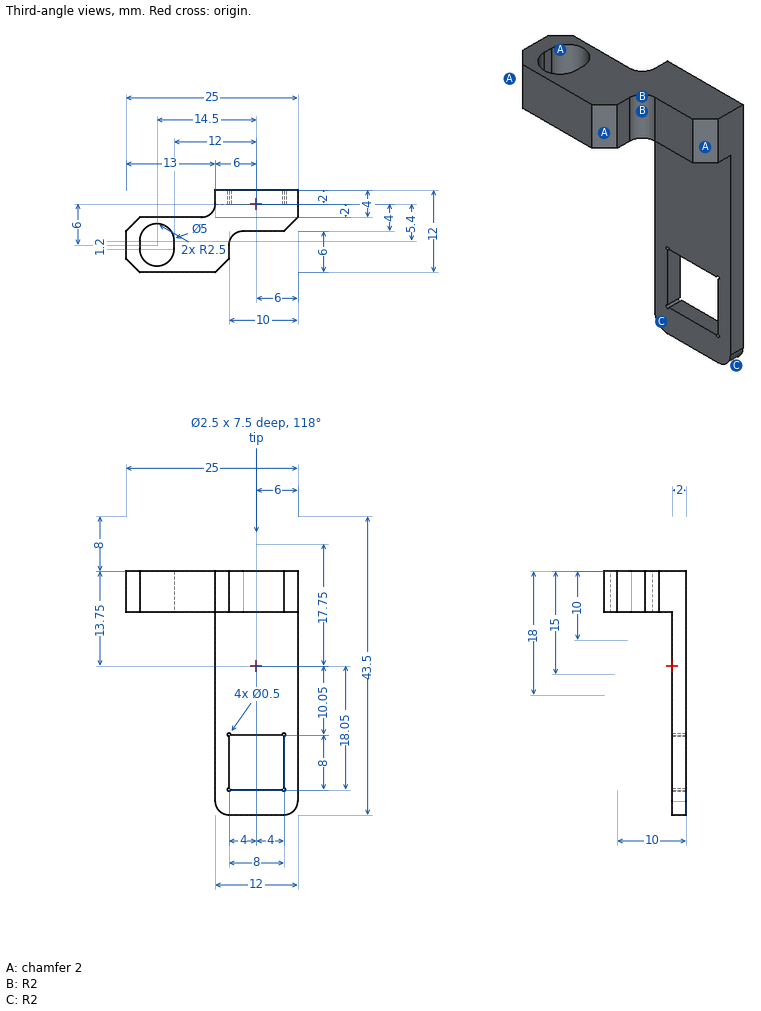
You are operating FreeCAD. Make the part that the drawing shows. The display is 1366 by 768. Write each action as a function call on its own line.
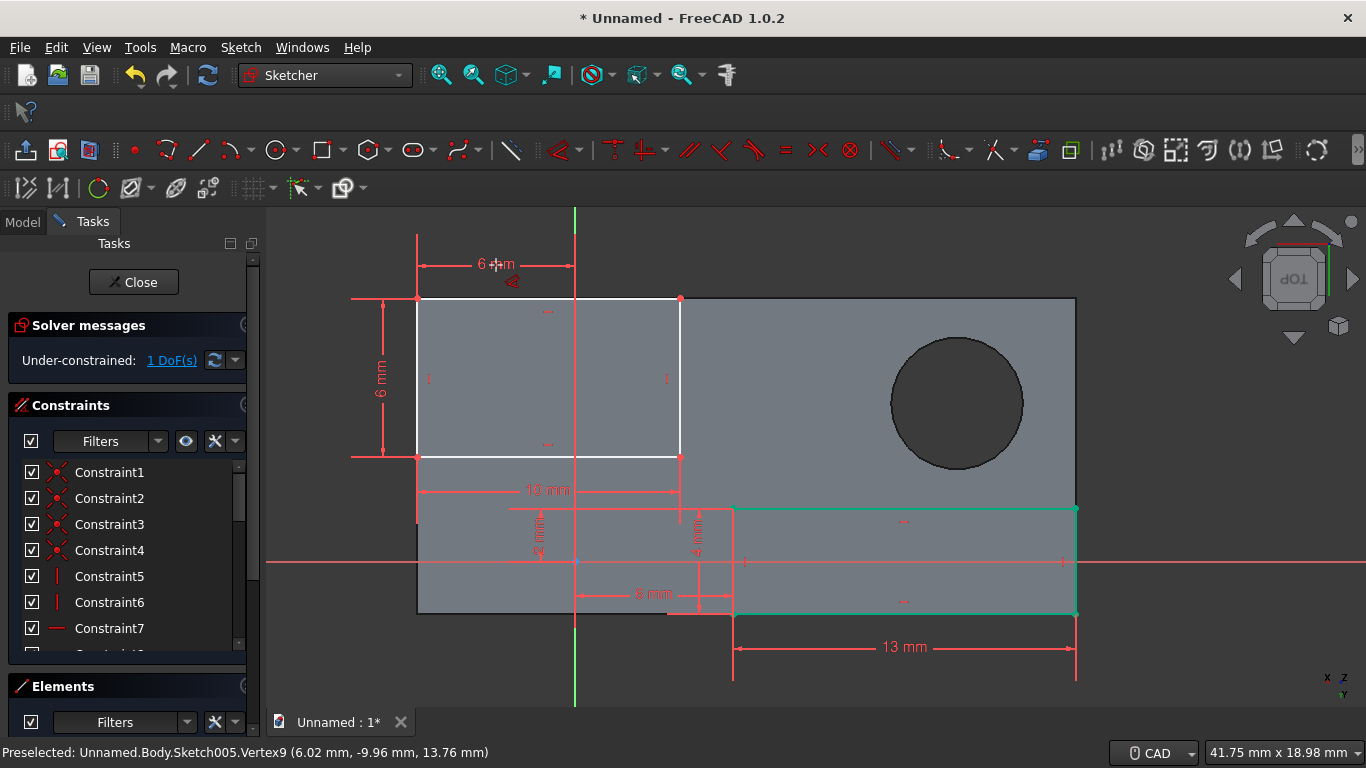
click(417, 457)
click(383, 509)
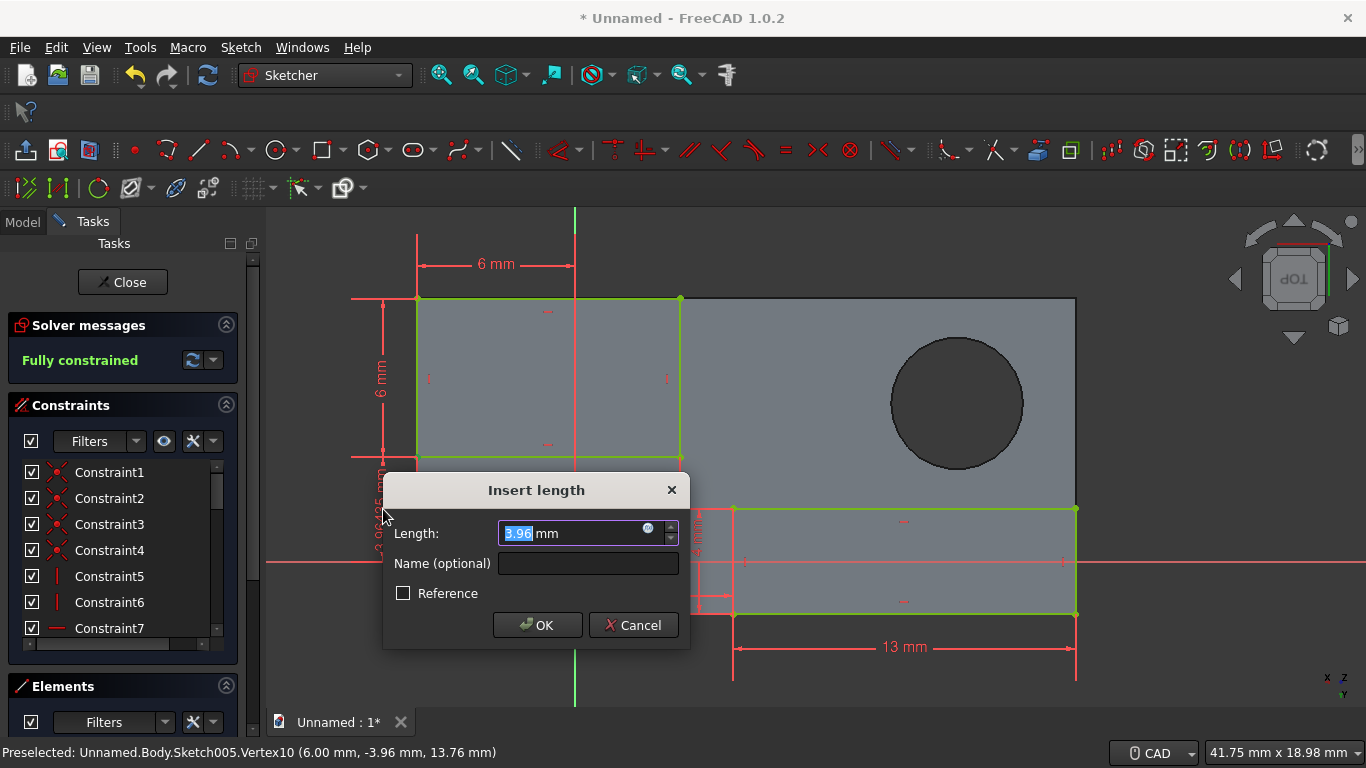
text(4)
key(Return)
key(Escape)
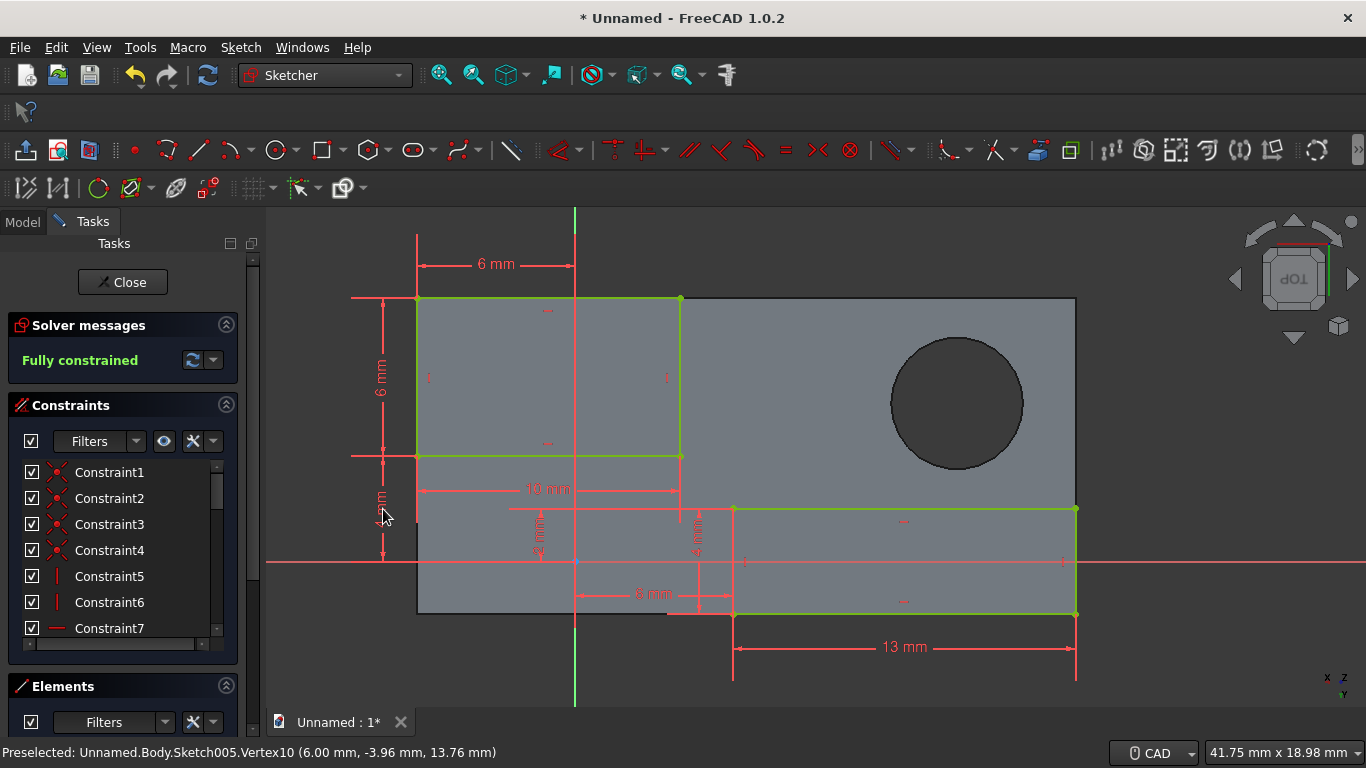
click(123, 282)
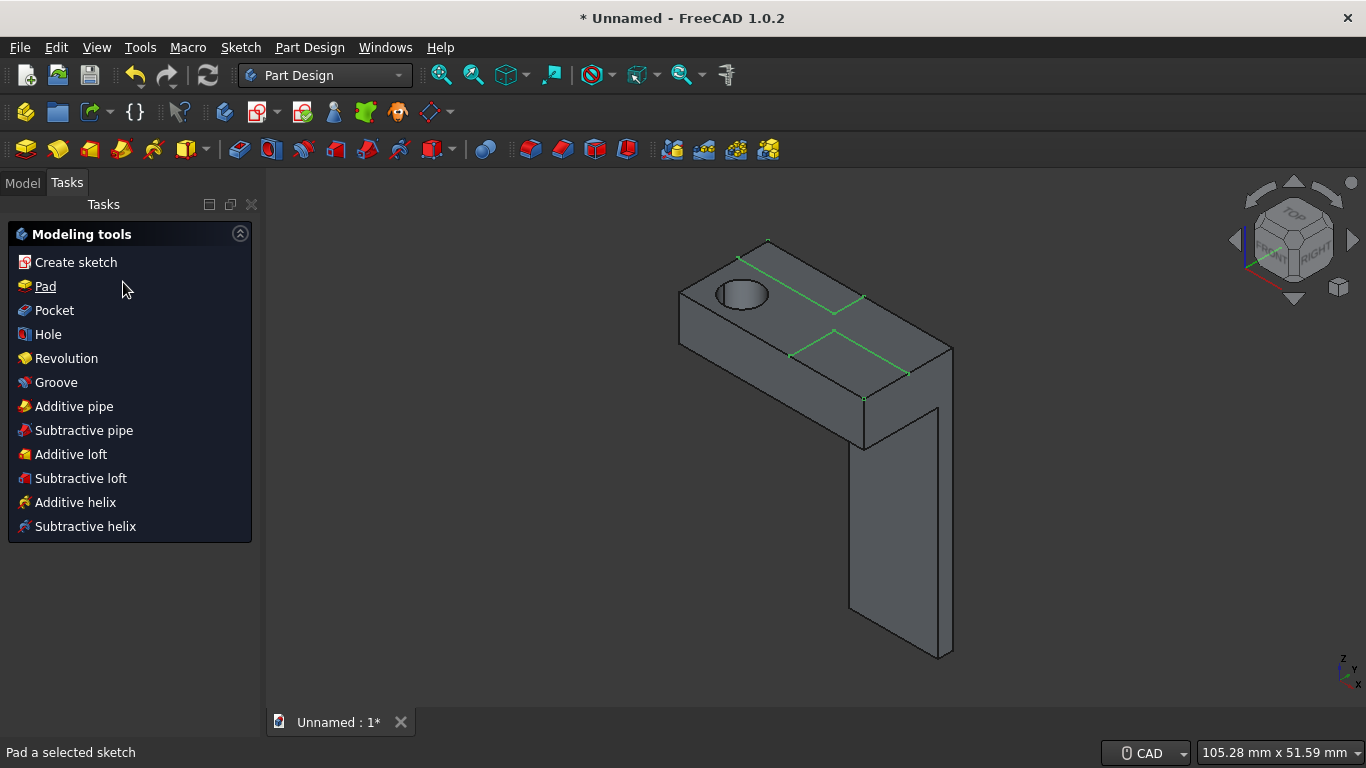
click(240, 150)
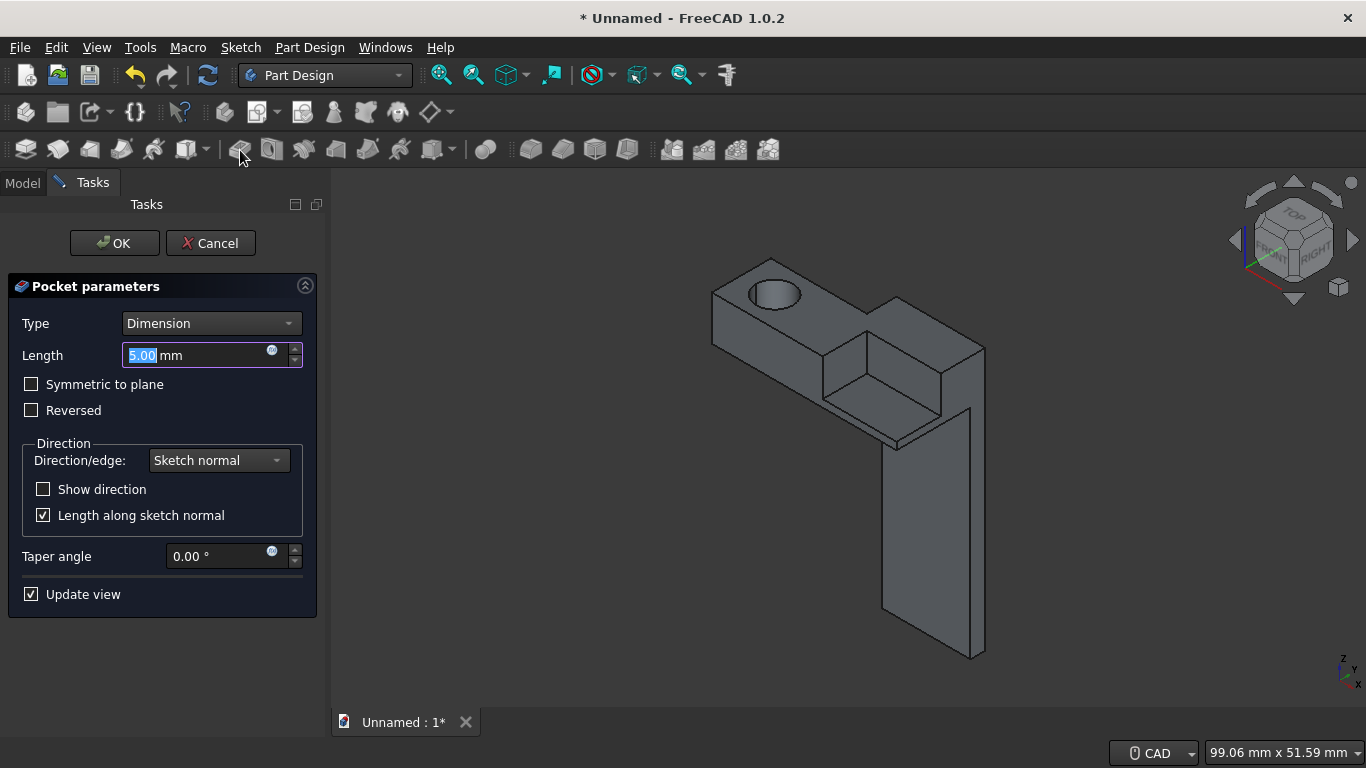
text(18)
key(Tab)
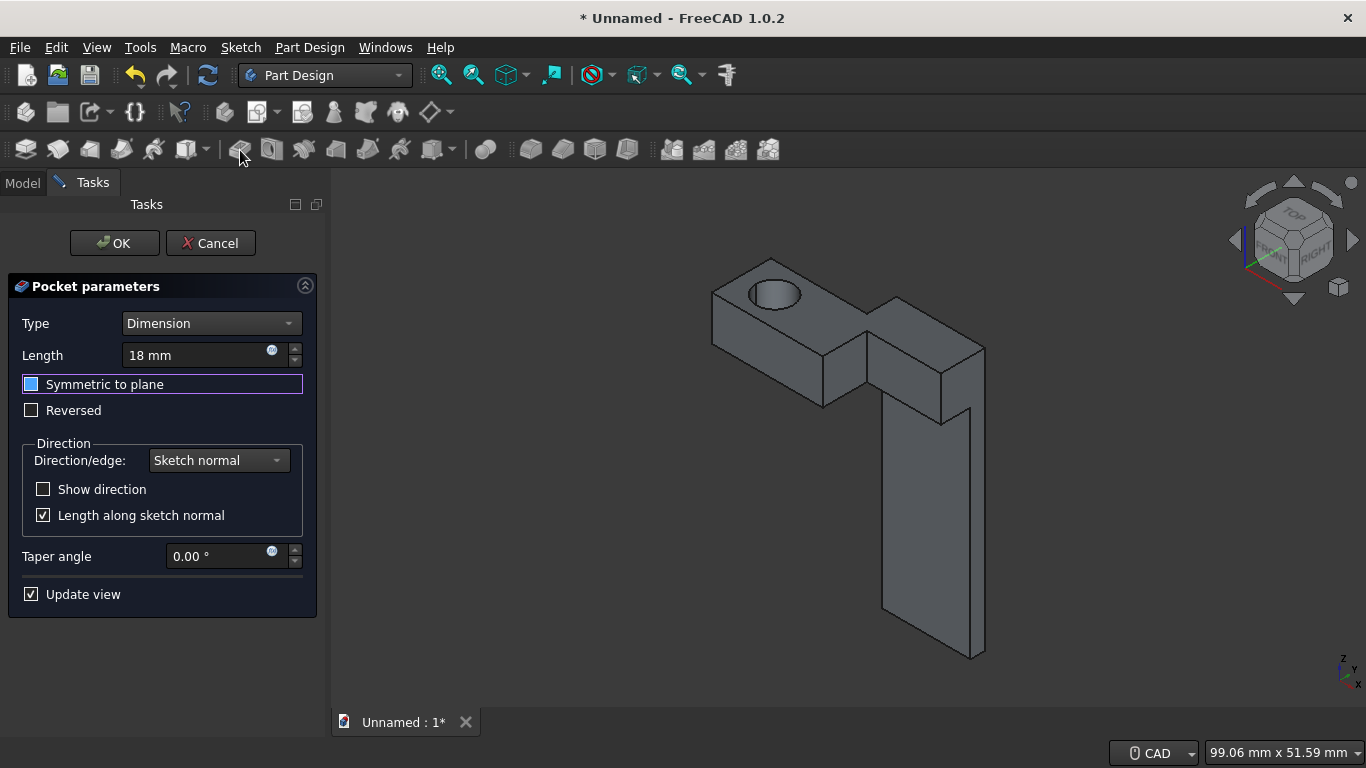
click(115, 243)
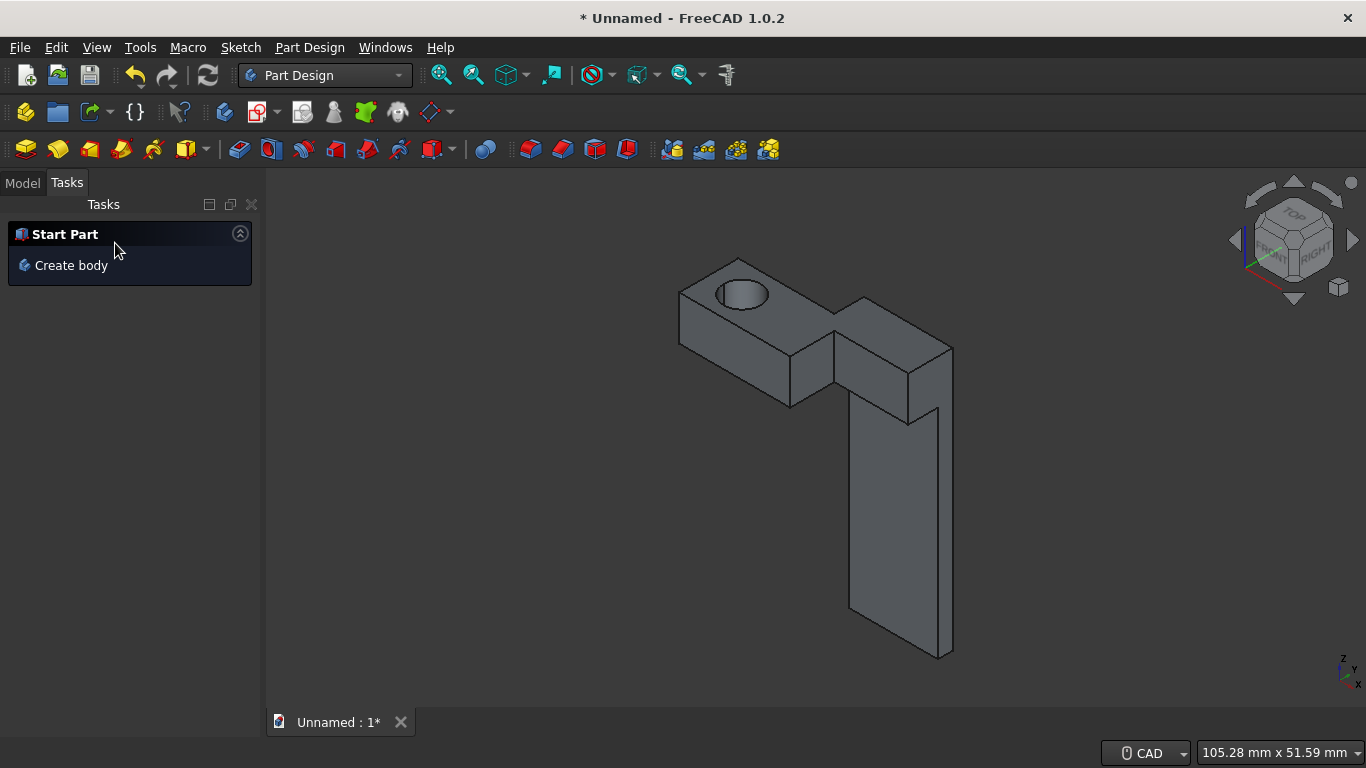
click(908, 398)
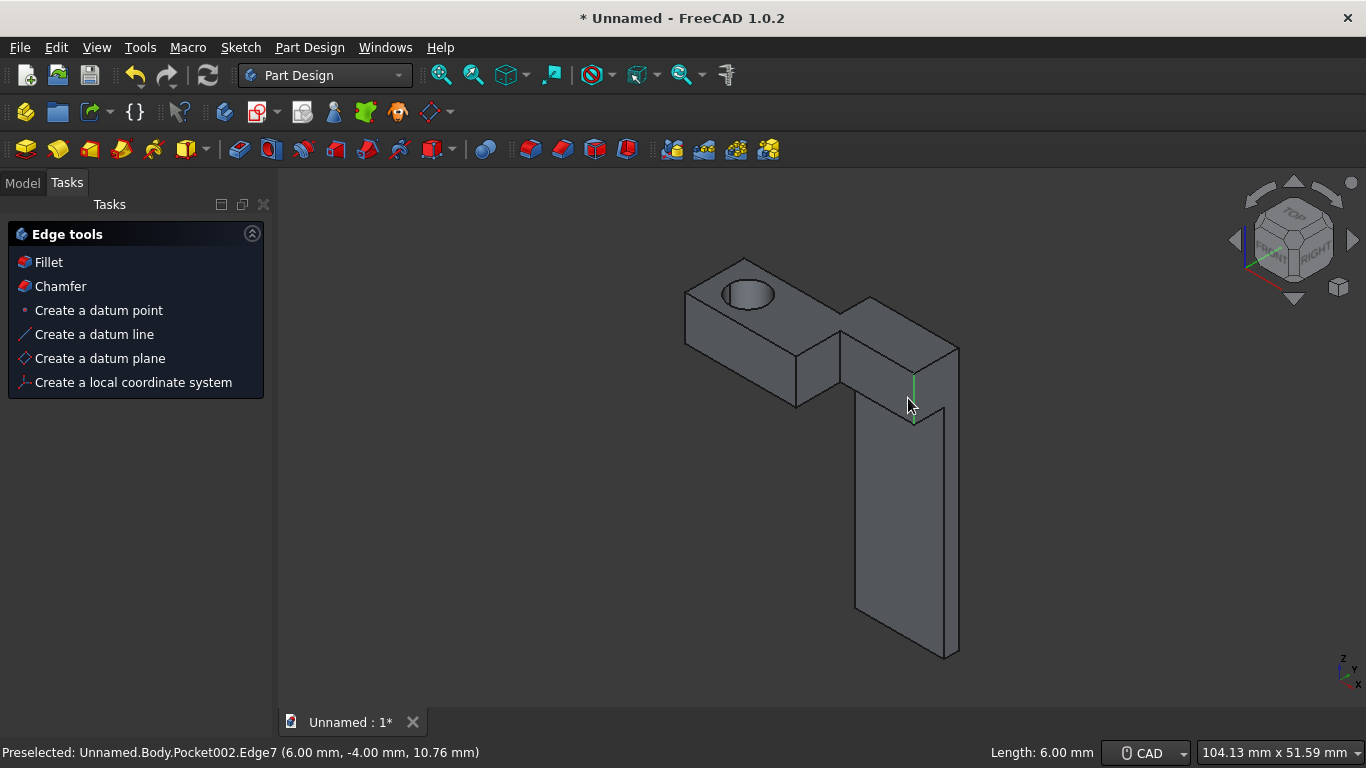
click(796, 381, ctrl)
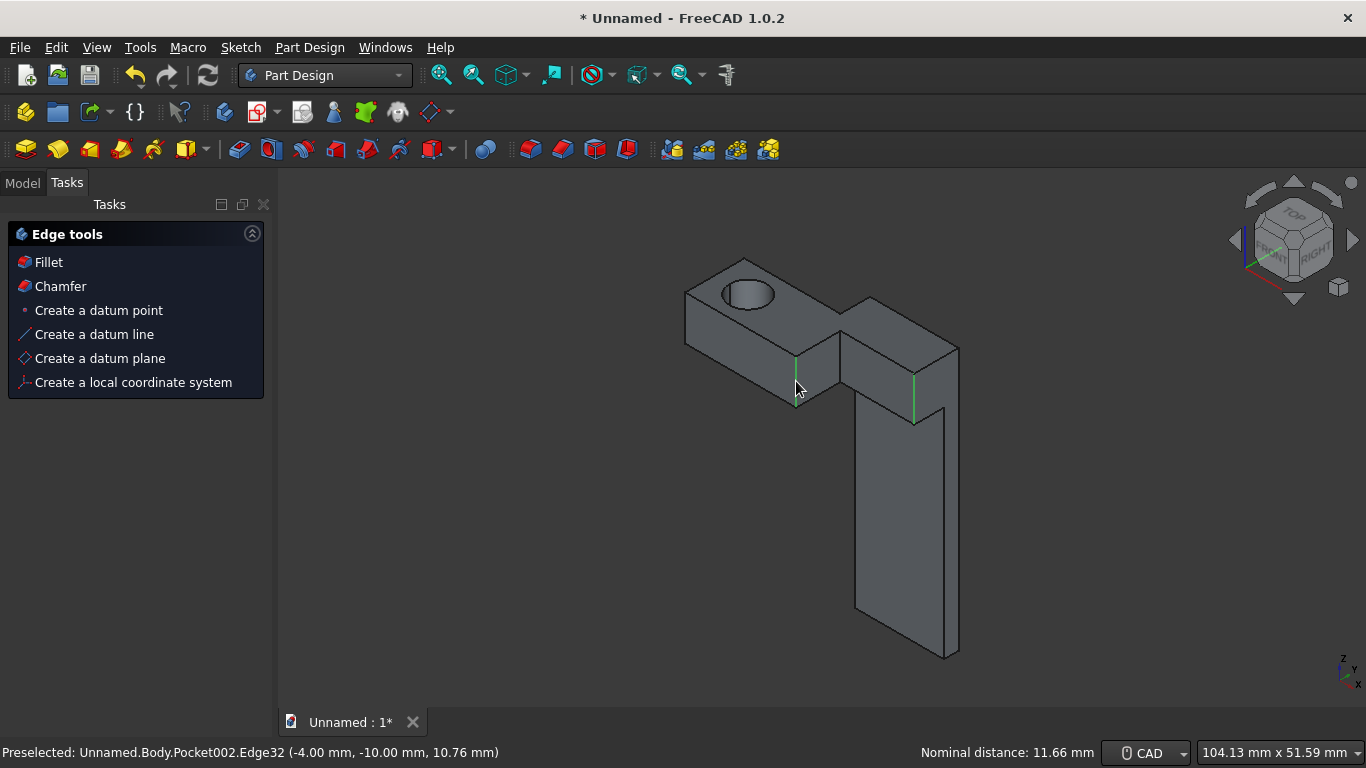
key(2)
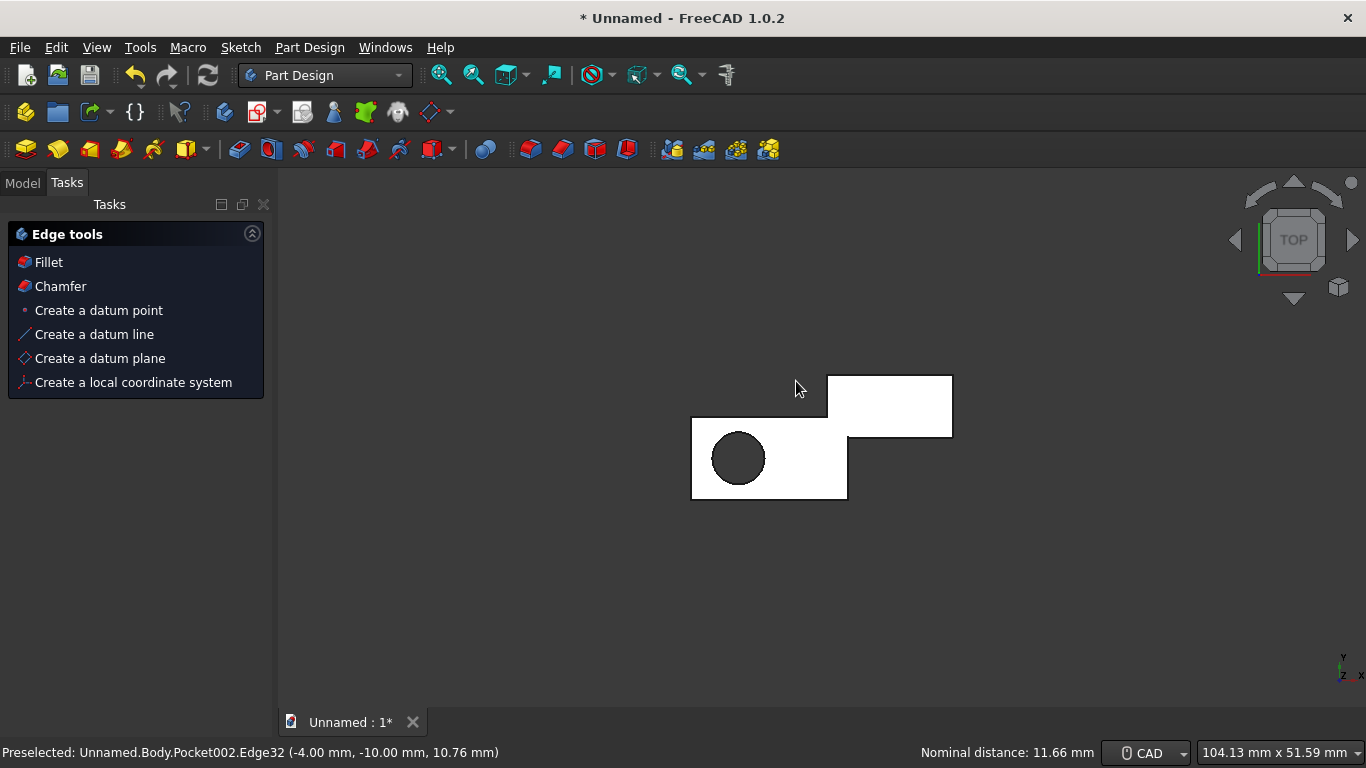
click(442, 76)